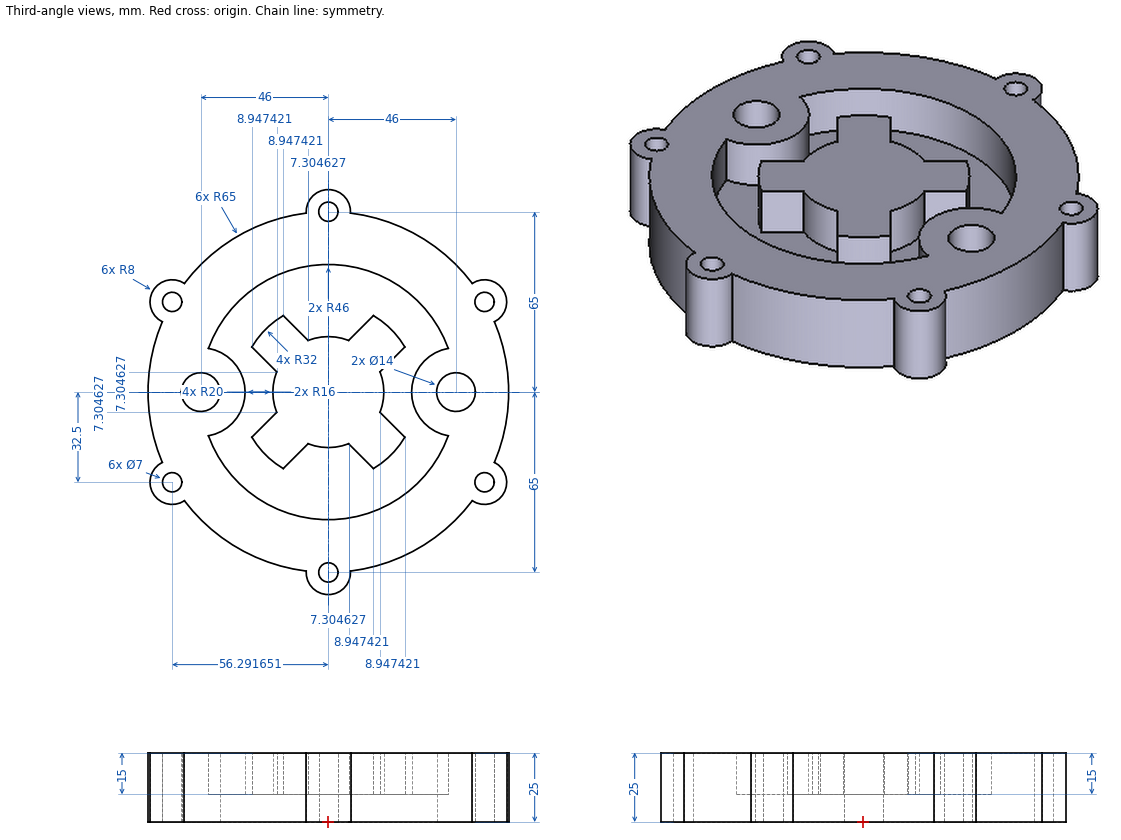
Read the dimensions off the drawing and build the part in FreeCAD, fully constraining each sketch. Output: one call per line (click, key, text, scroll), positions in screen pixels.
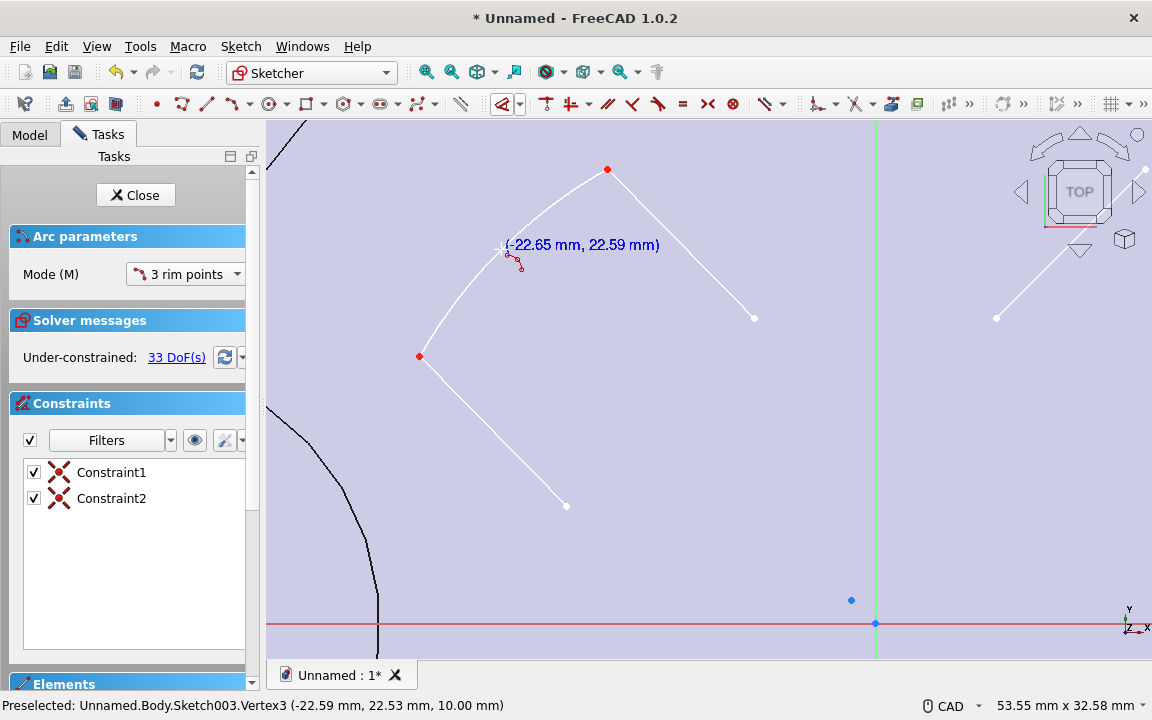
click(567, 506)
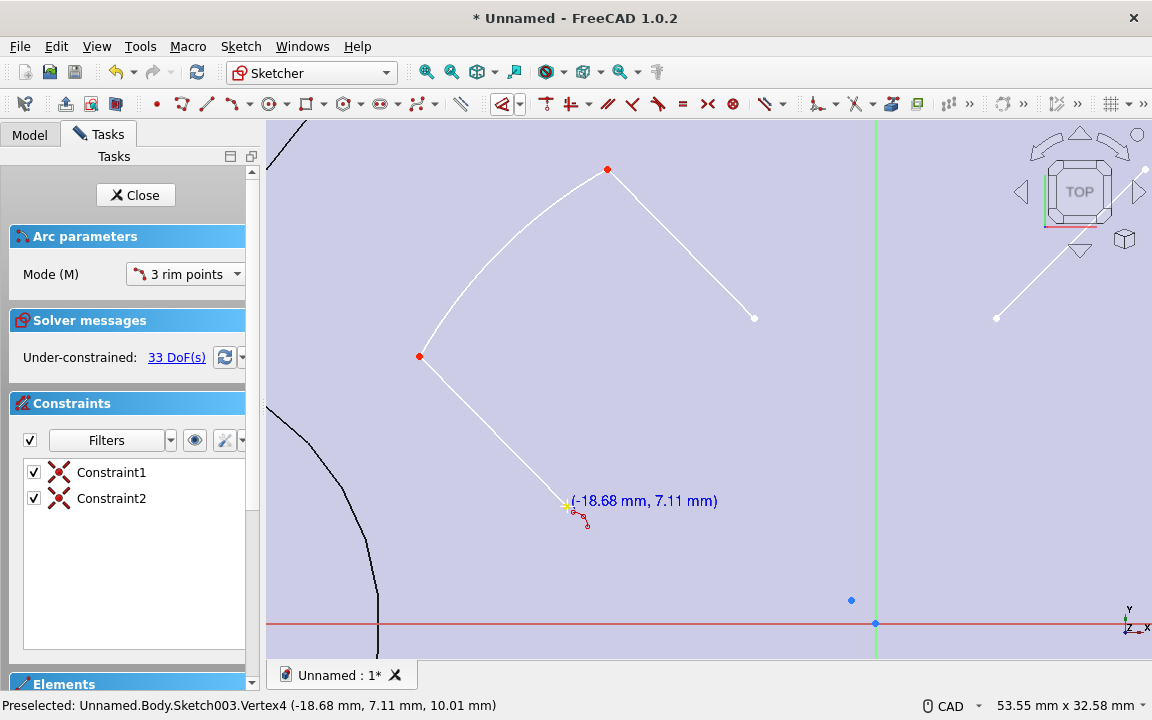
scroll(504, 253, down, 5)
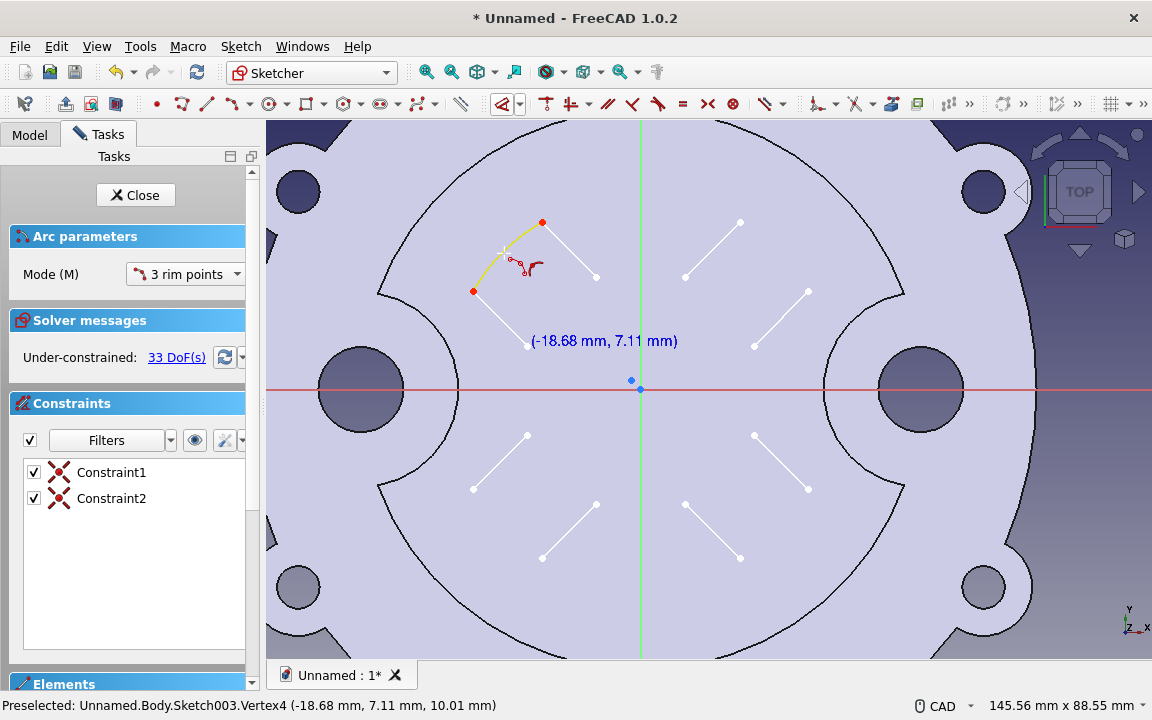
click(527, 435)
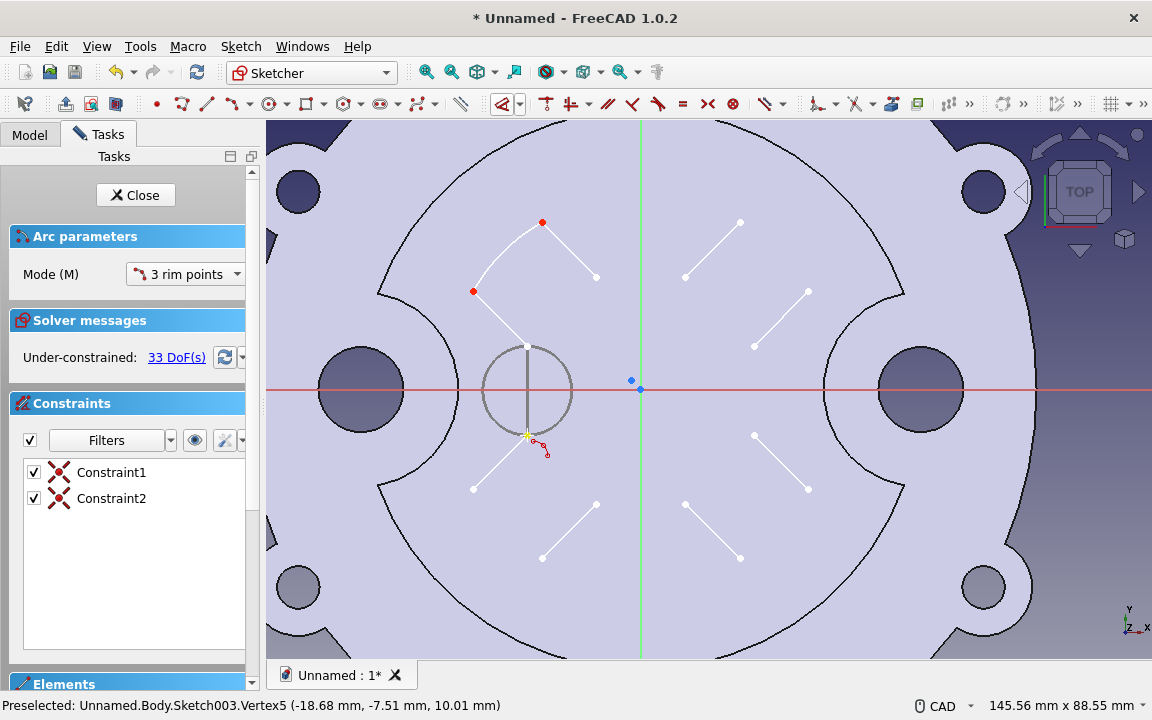
scroll(520, 380, up, 4)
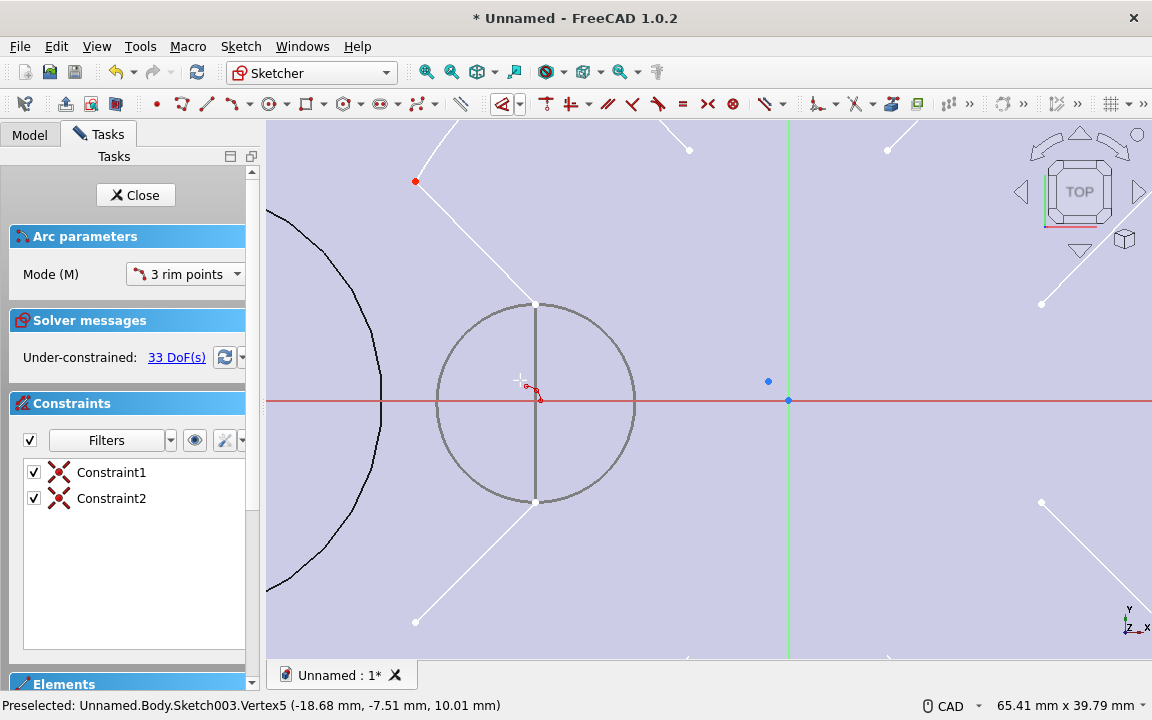
click(519, 380)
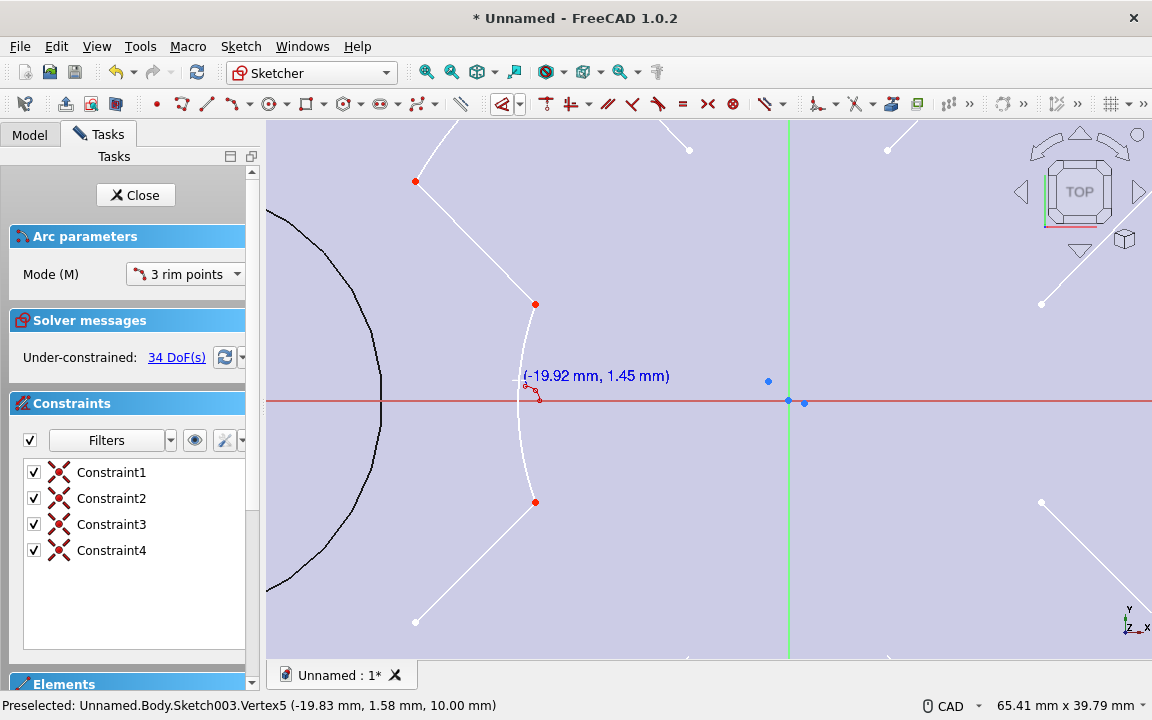
click(416, 623)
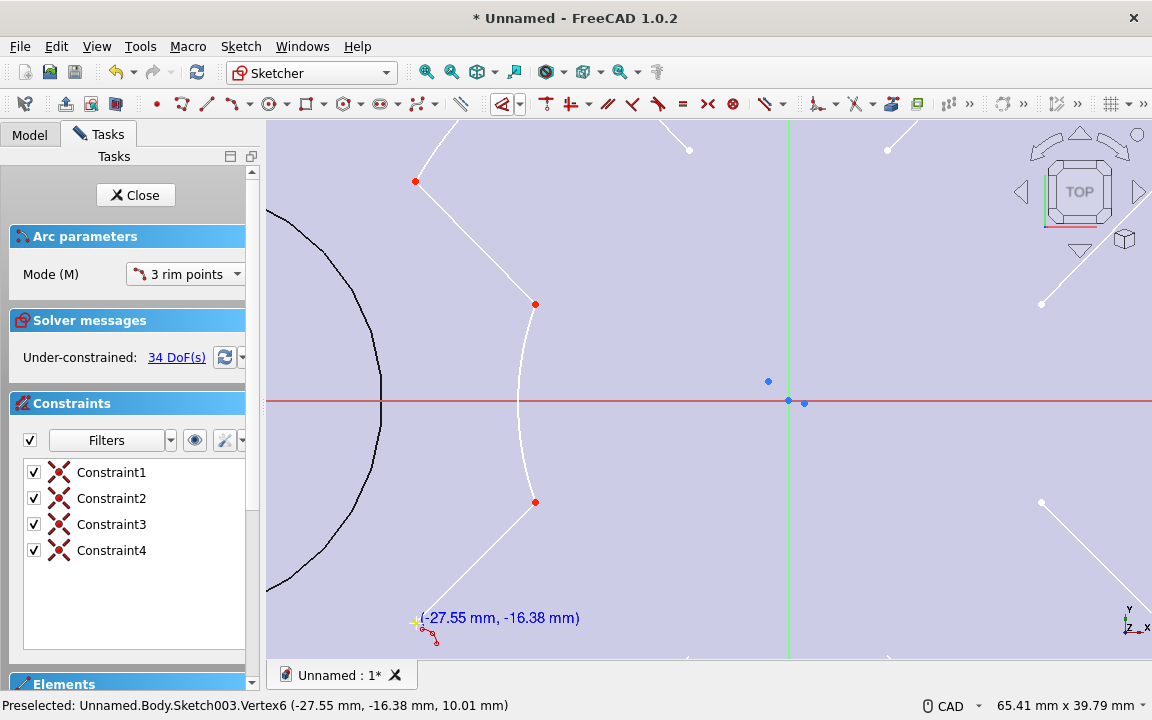
scroll(519, 380, down, 4)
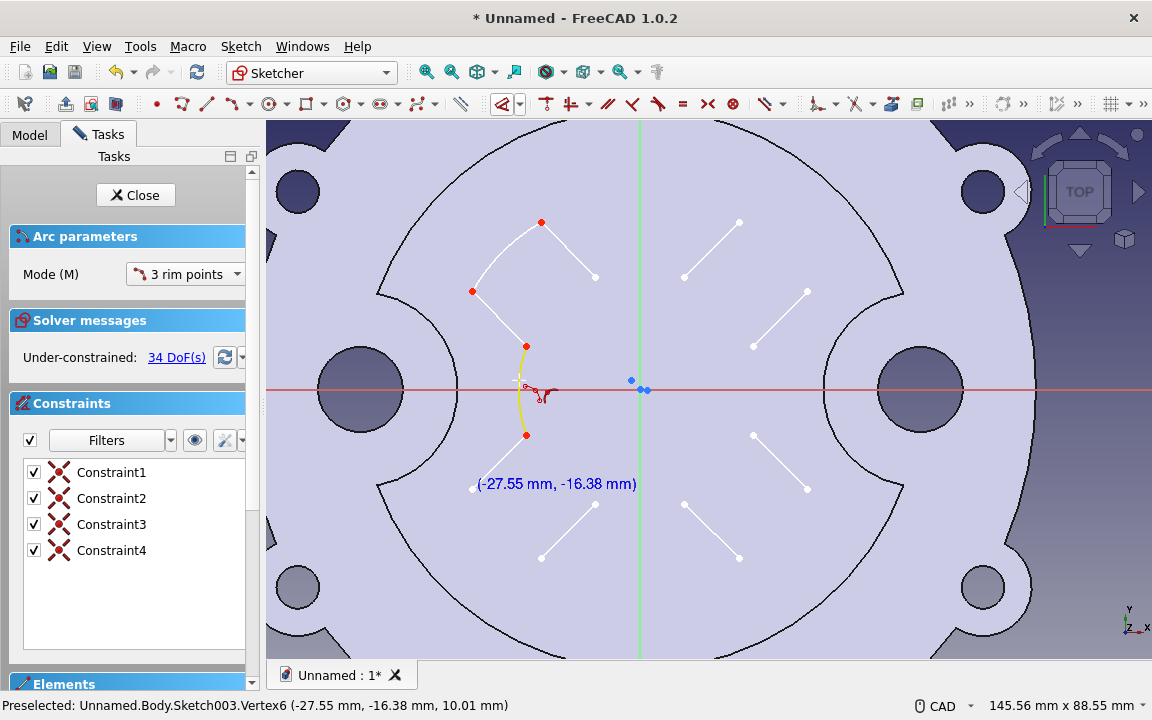
click(542, 558)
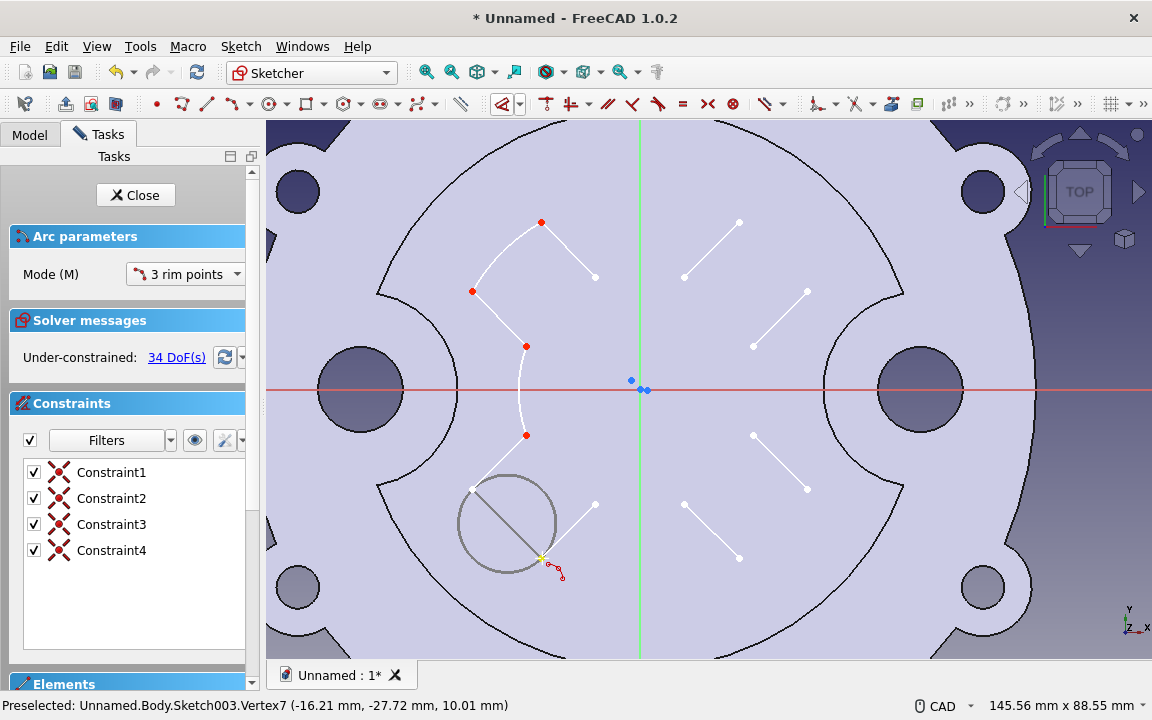
scroll(503, 527, up, 5)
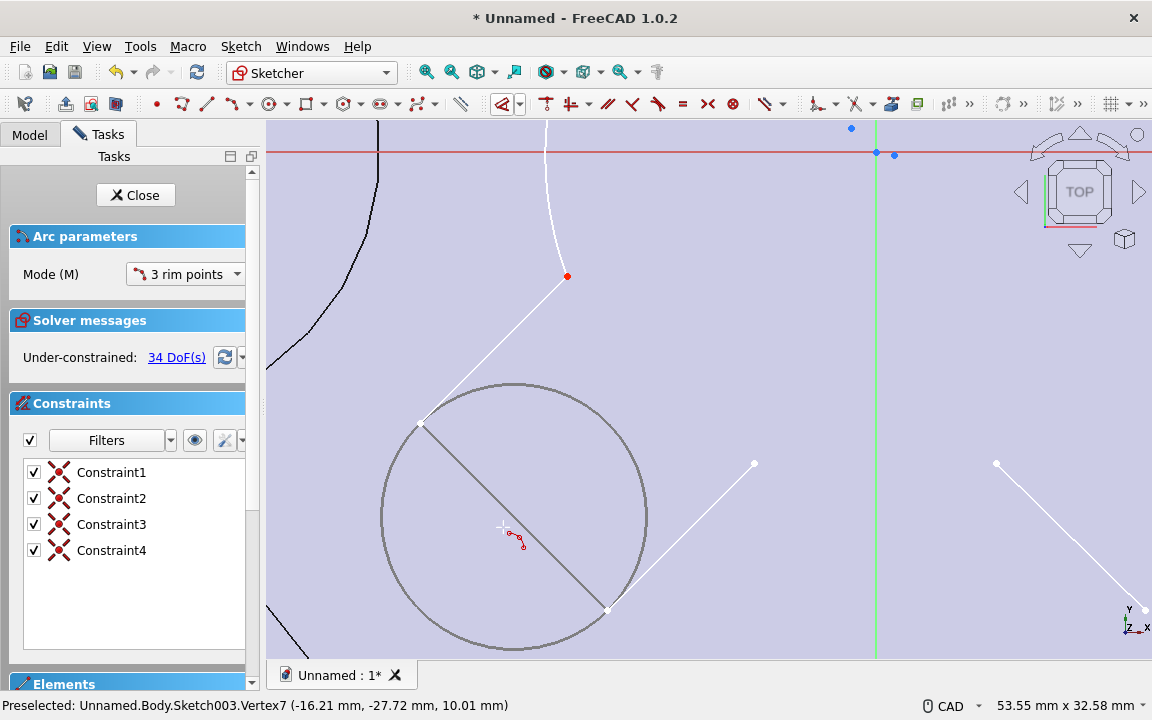
click(502, 526)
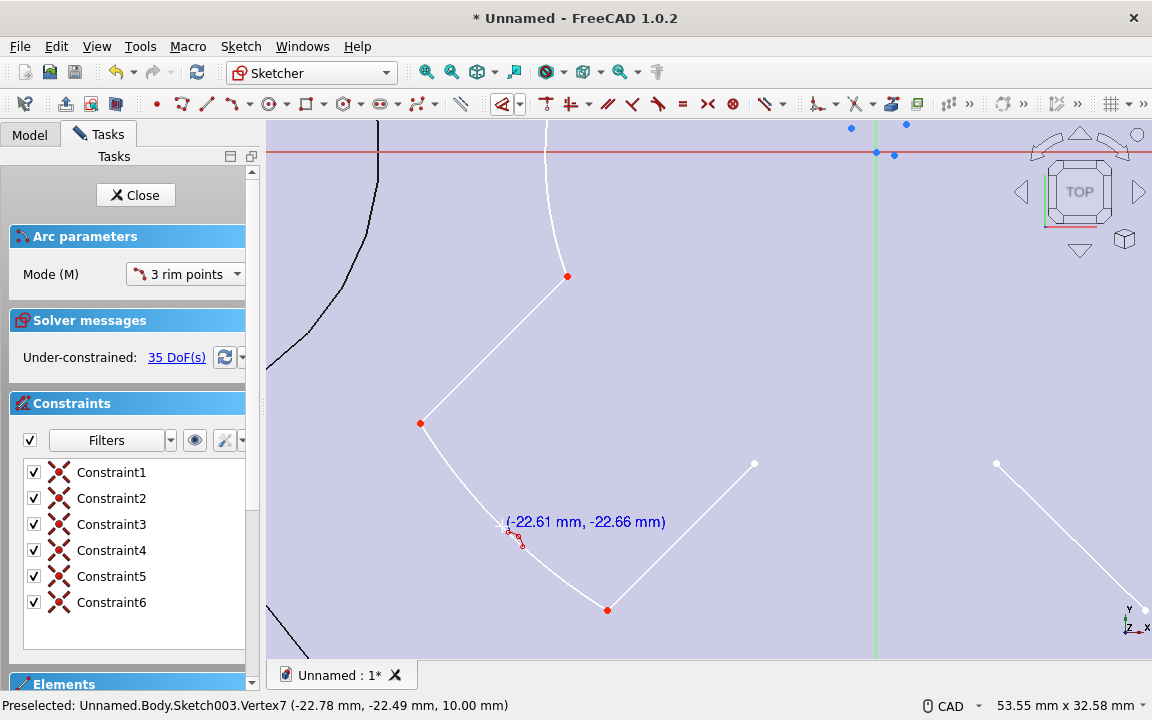
click(755, 464)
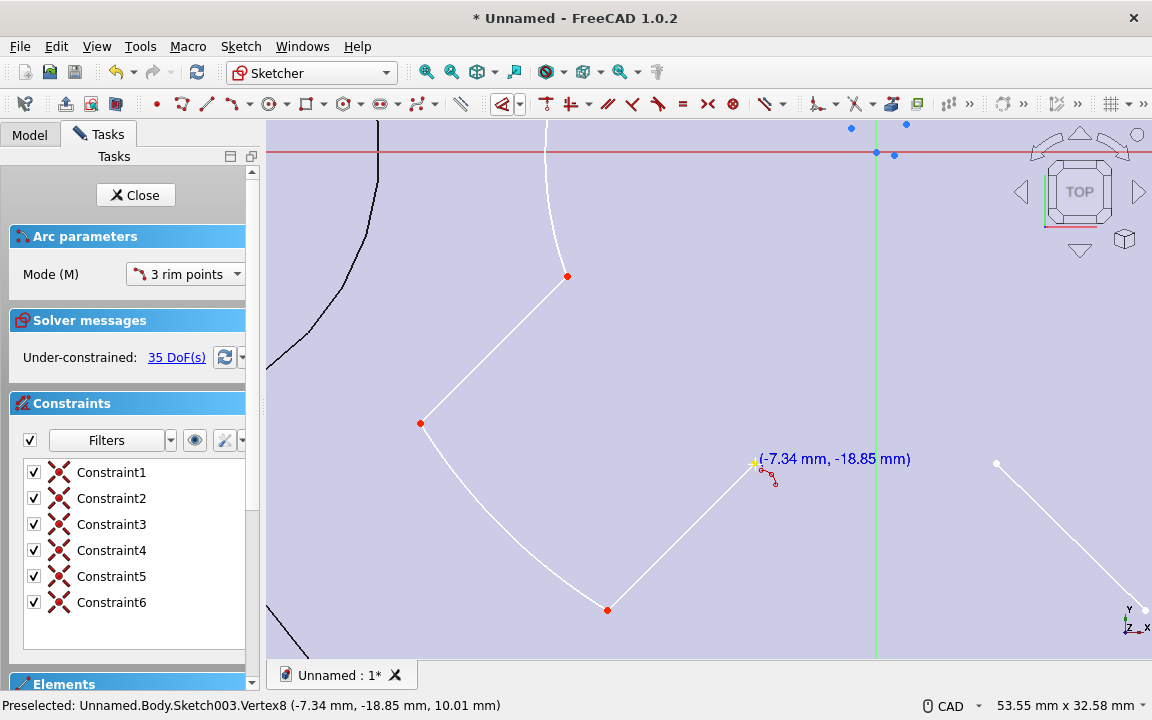
scroll(503, 528, down, 5)